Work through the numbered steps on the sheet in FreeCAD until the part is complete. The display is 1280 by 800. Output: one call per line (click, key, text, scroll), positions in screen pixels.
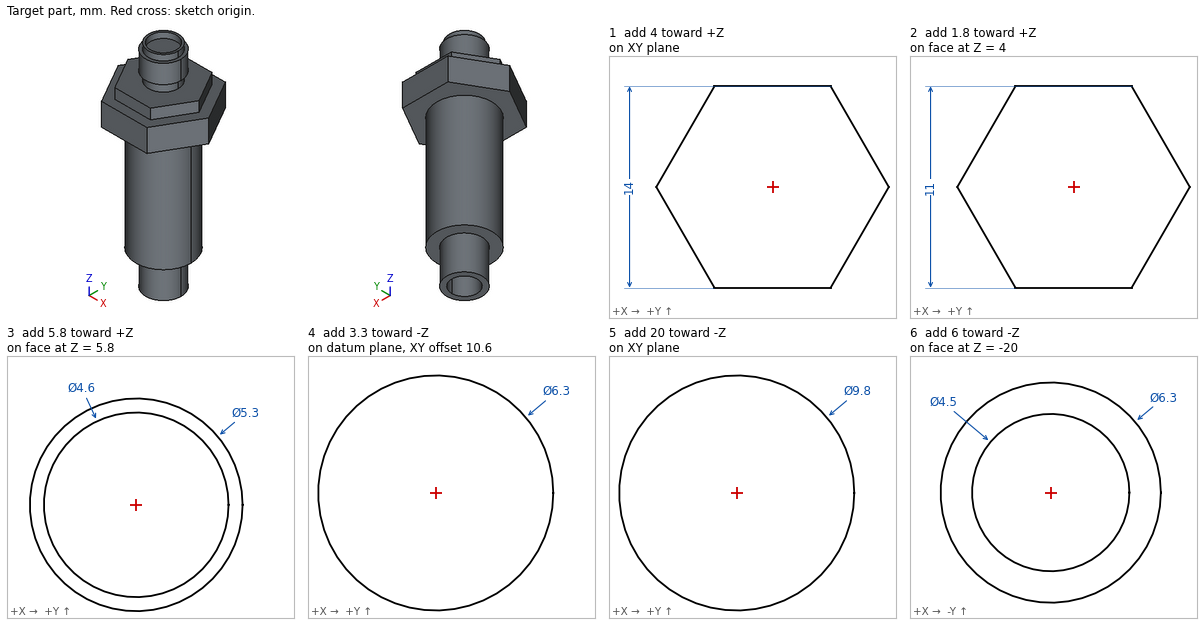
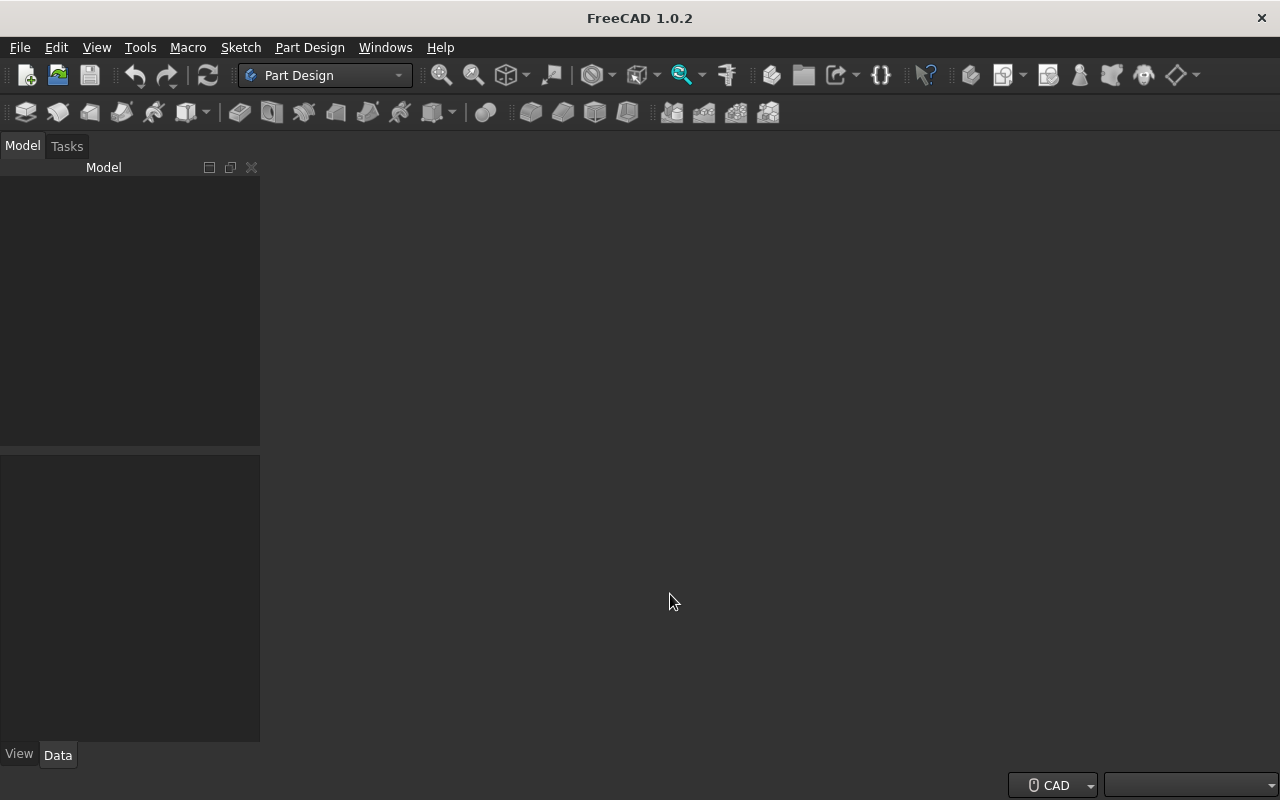
key(ctrl+n)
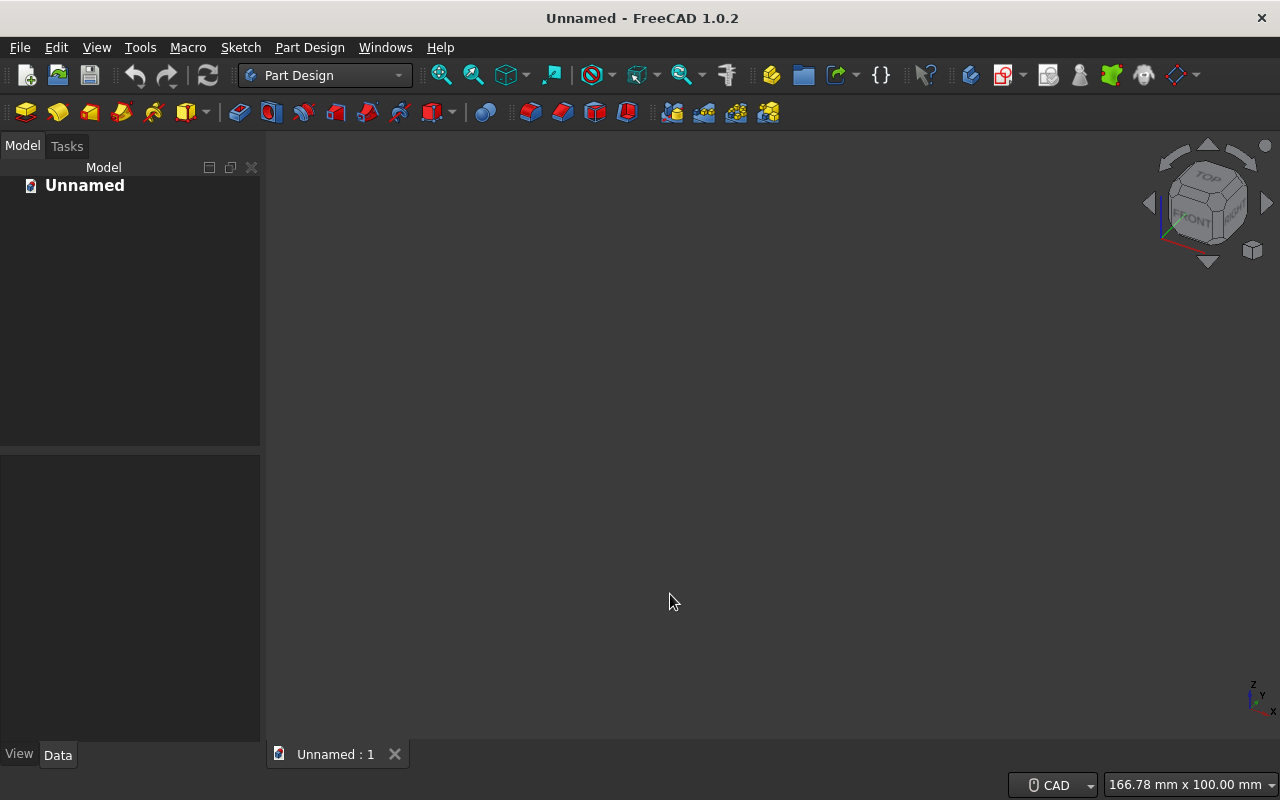
click(1004, 76)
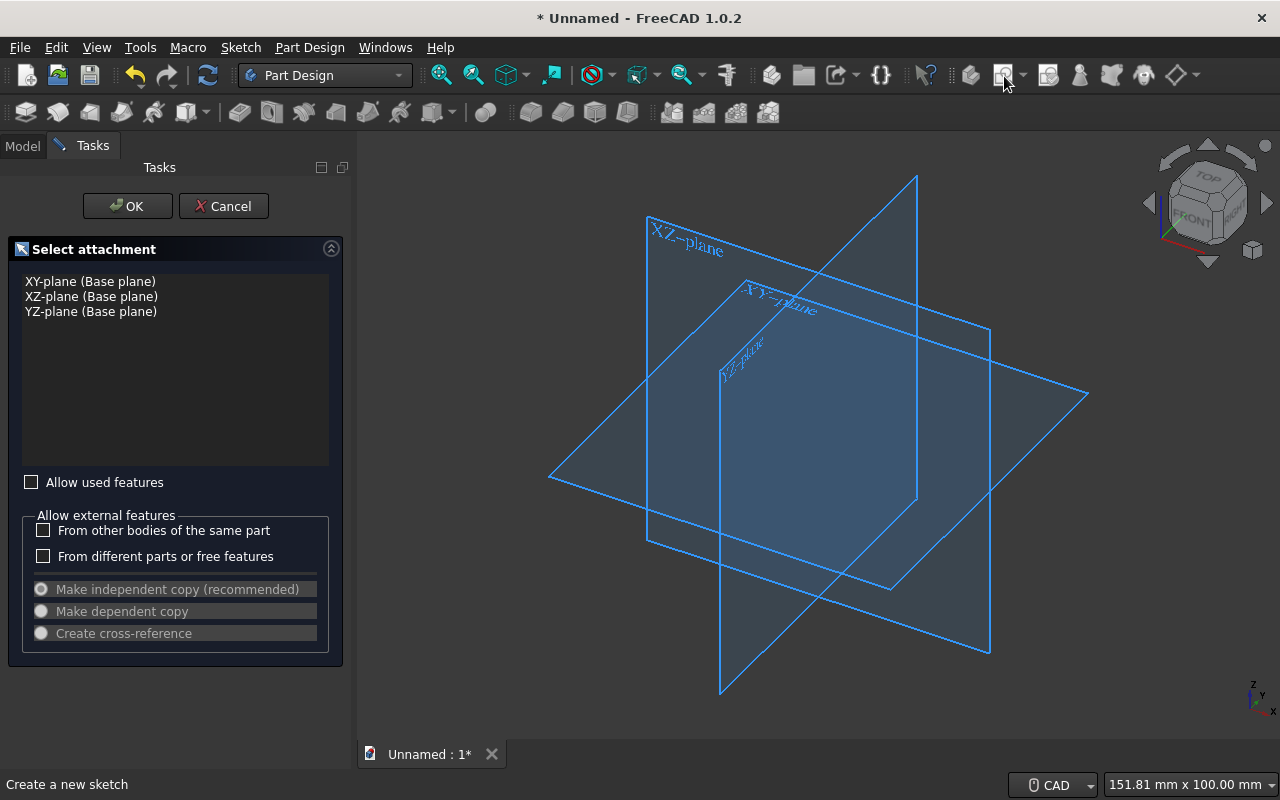
click(82, 282)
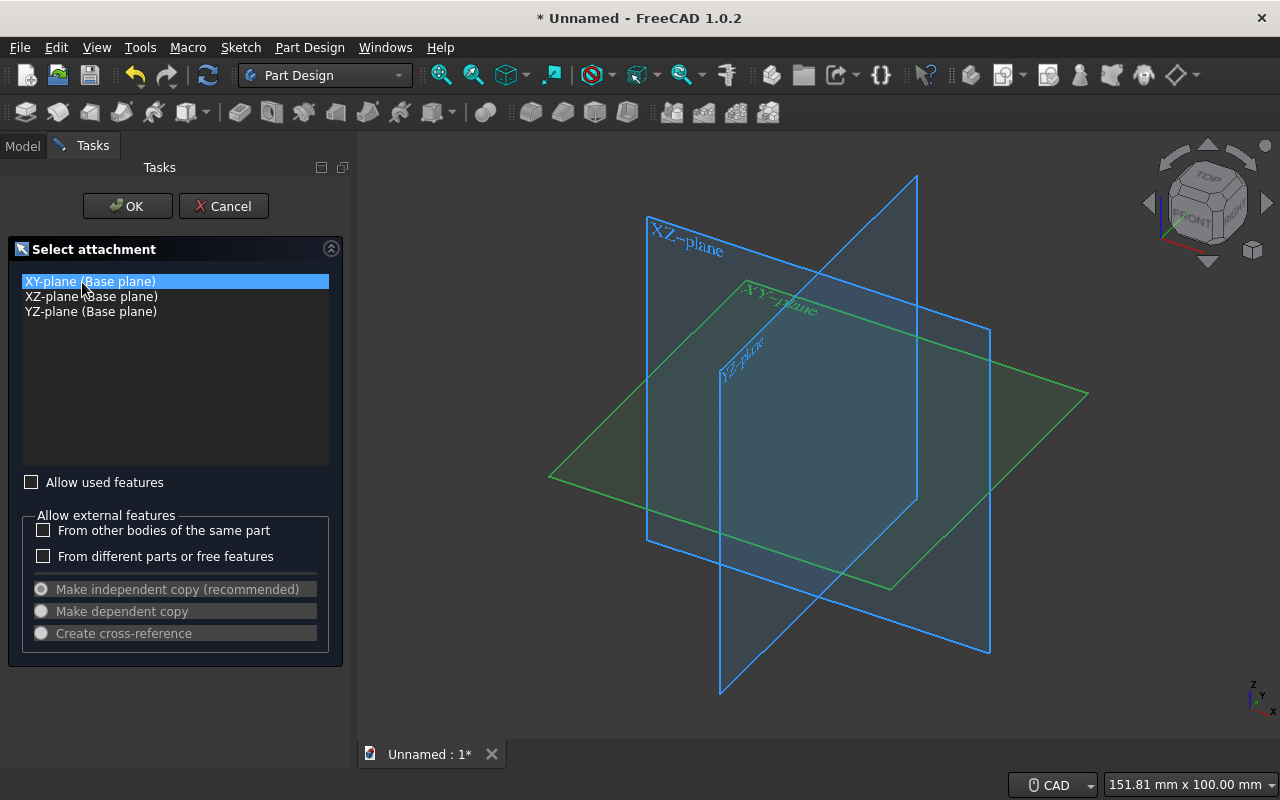
click(128, 206)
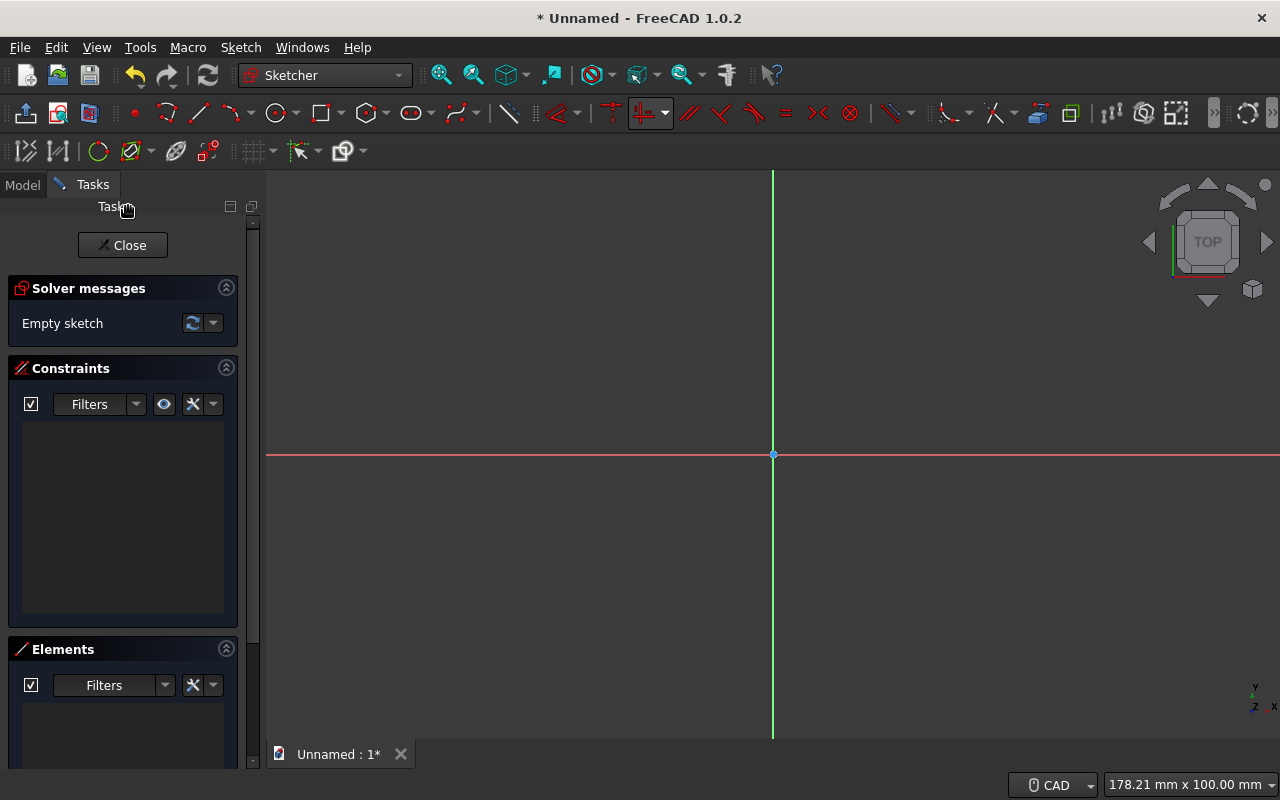
scroll(790, 454, up, 8)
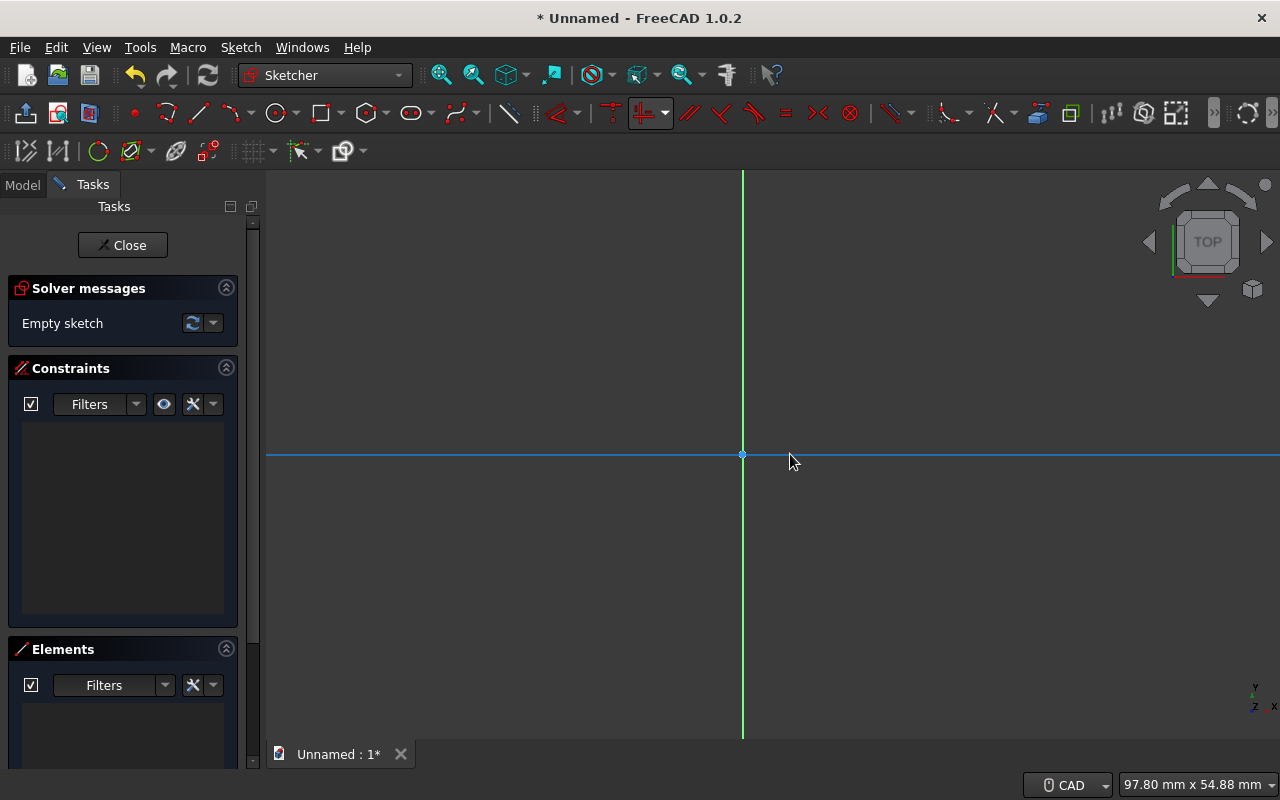
click(366, 114)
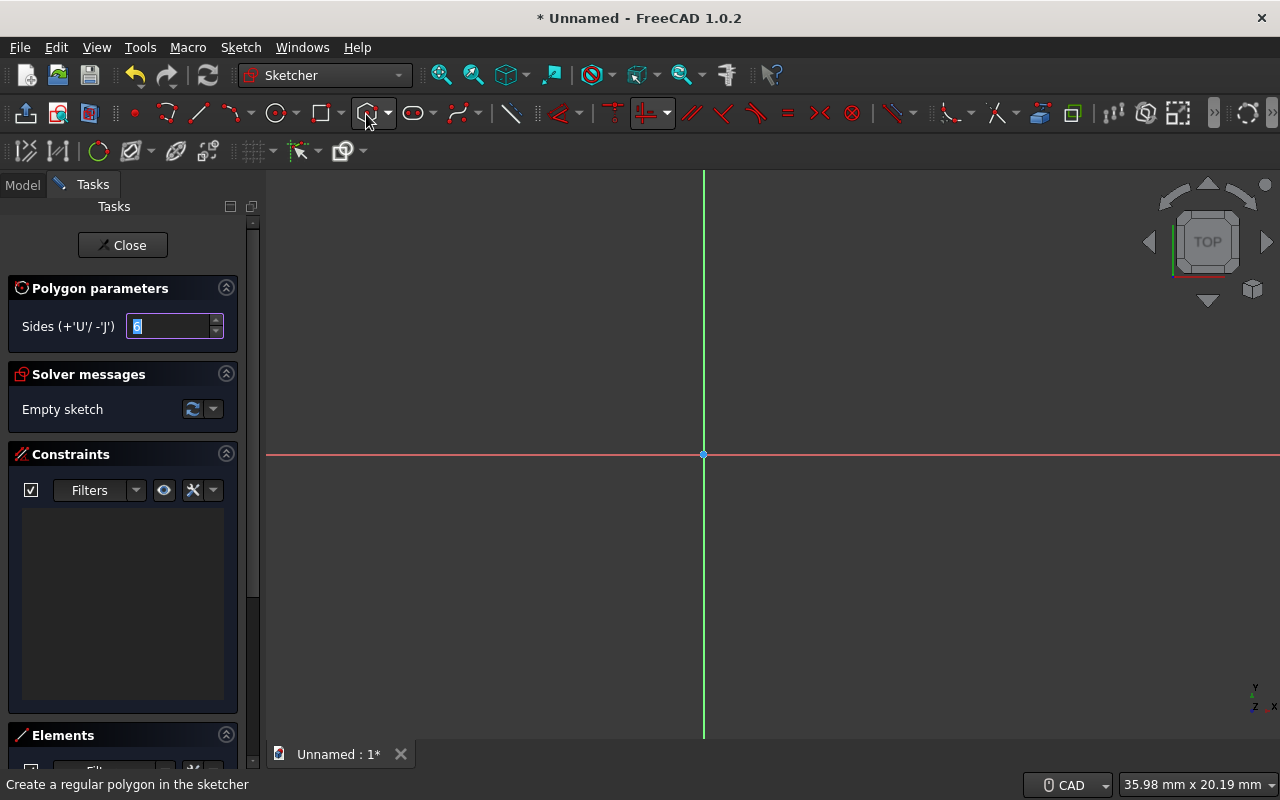
click(704, 454)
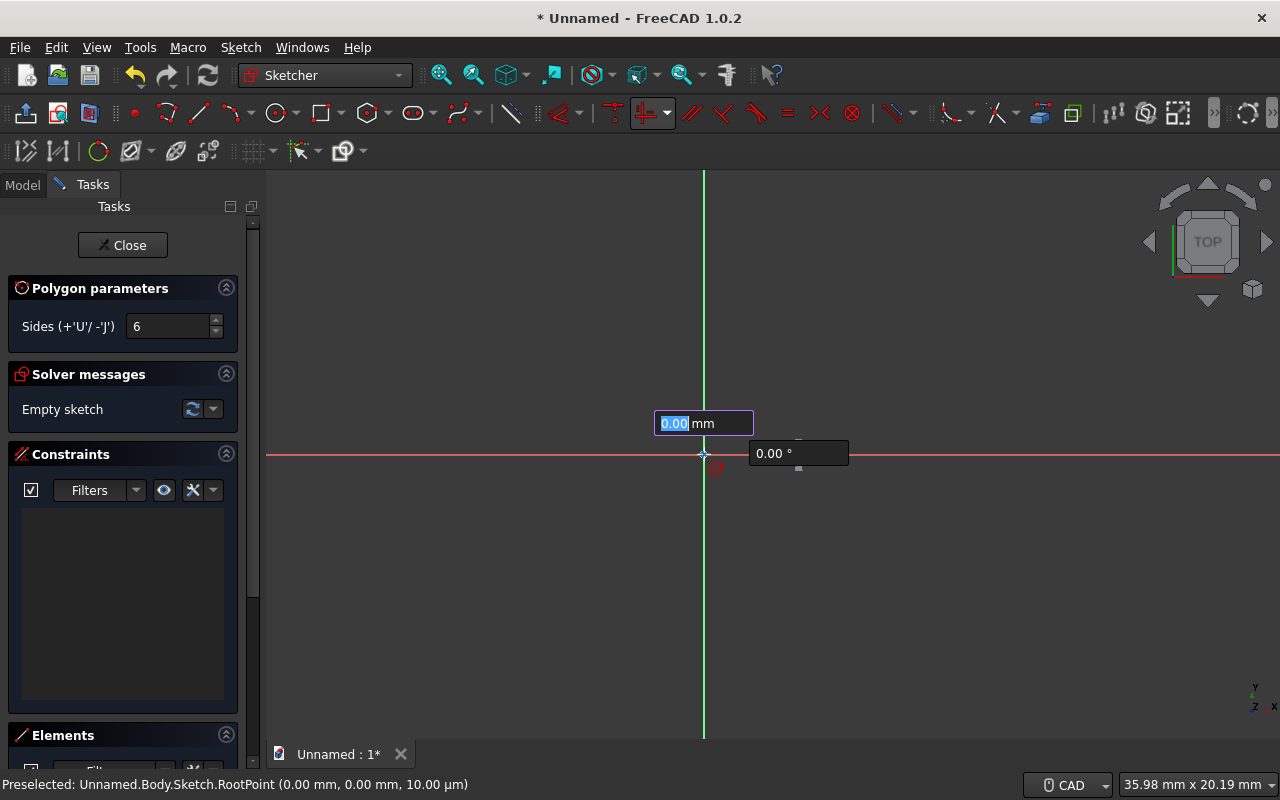
click(932, 454)
right_click(932, 454)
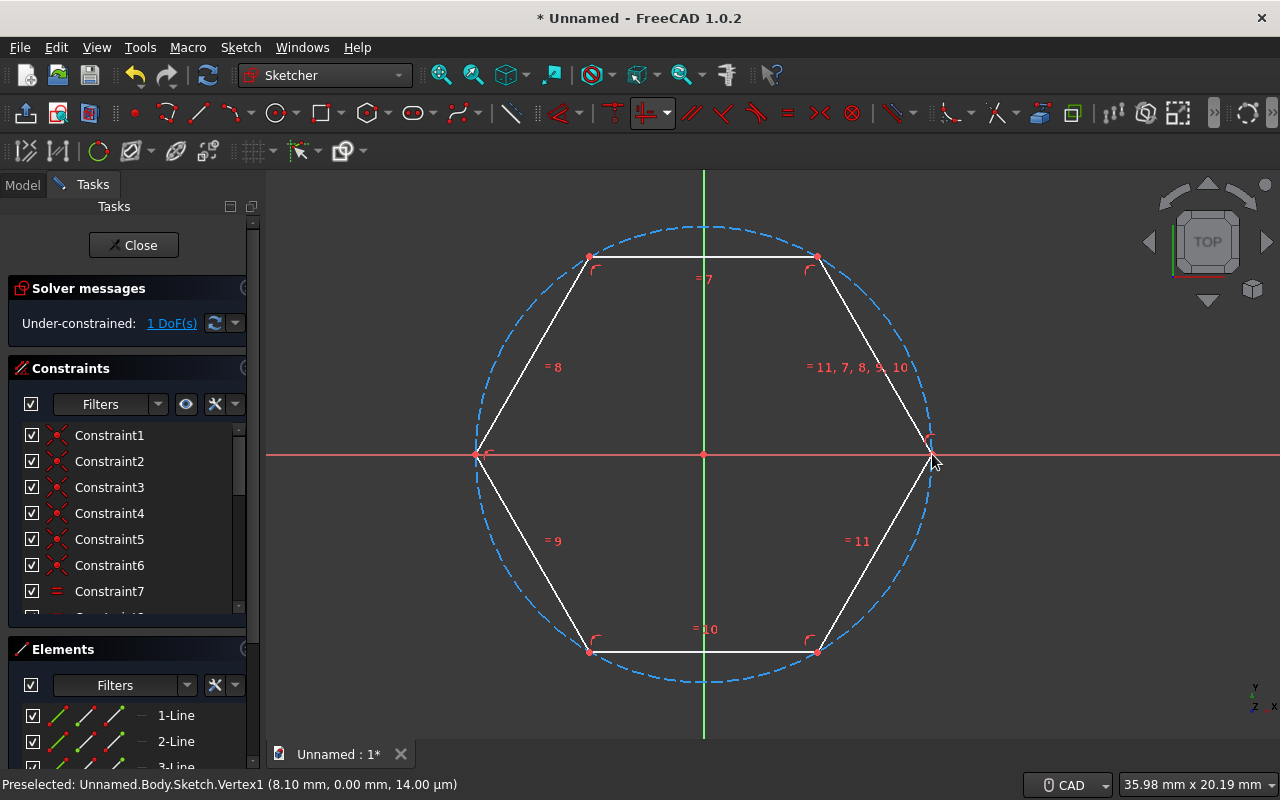
click(590, 652)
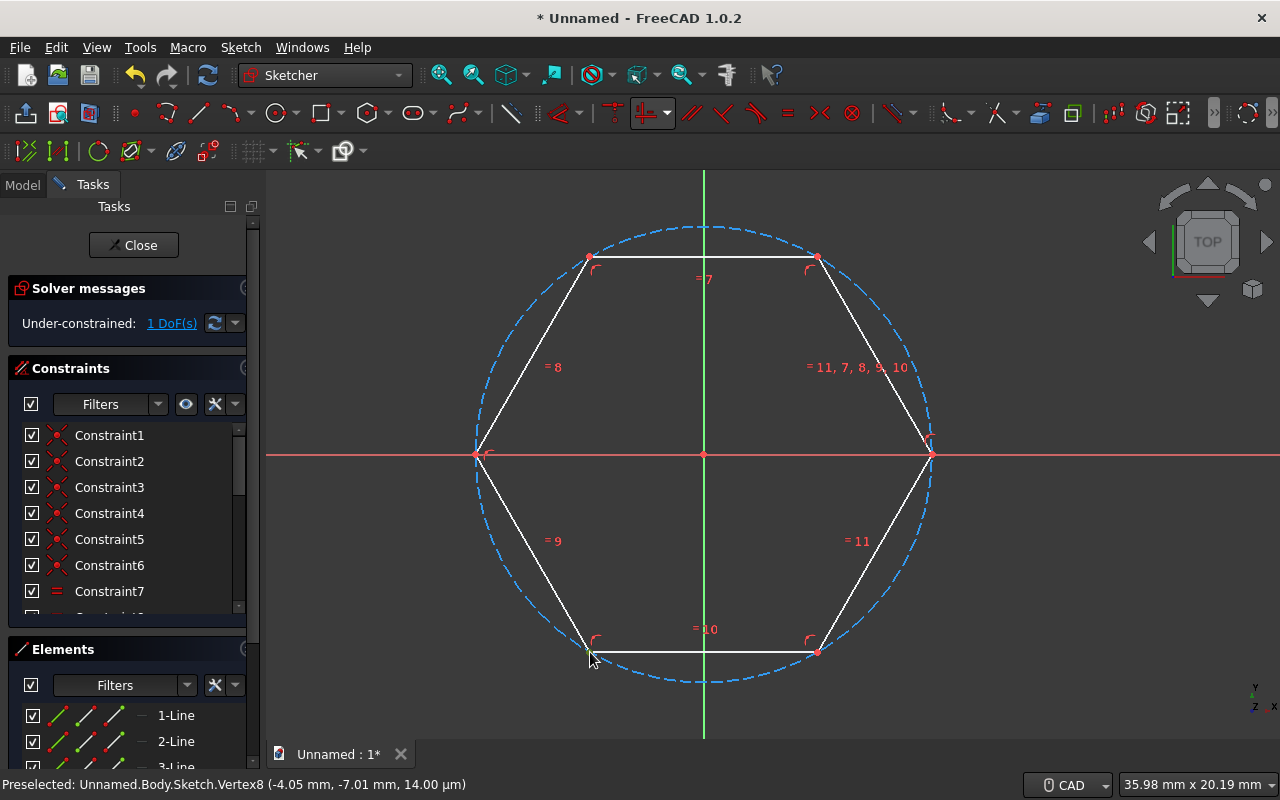
click(818, 257)